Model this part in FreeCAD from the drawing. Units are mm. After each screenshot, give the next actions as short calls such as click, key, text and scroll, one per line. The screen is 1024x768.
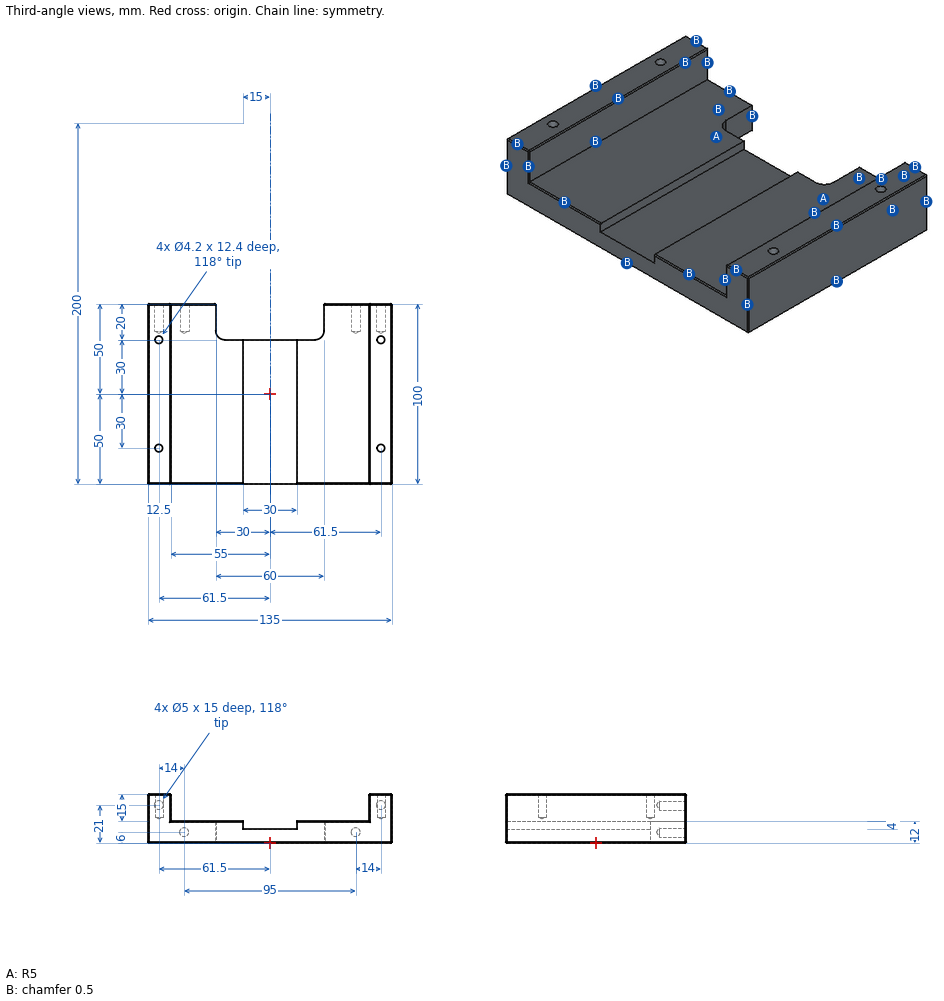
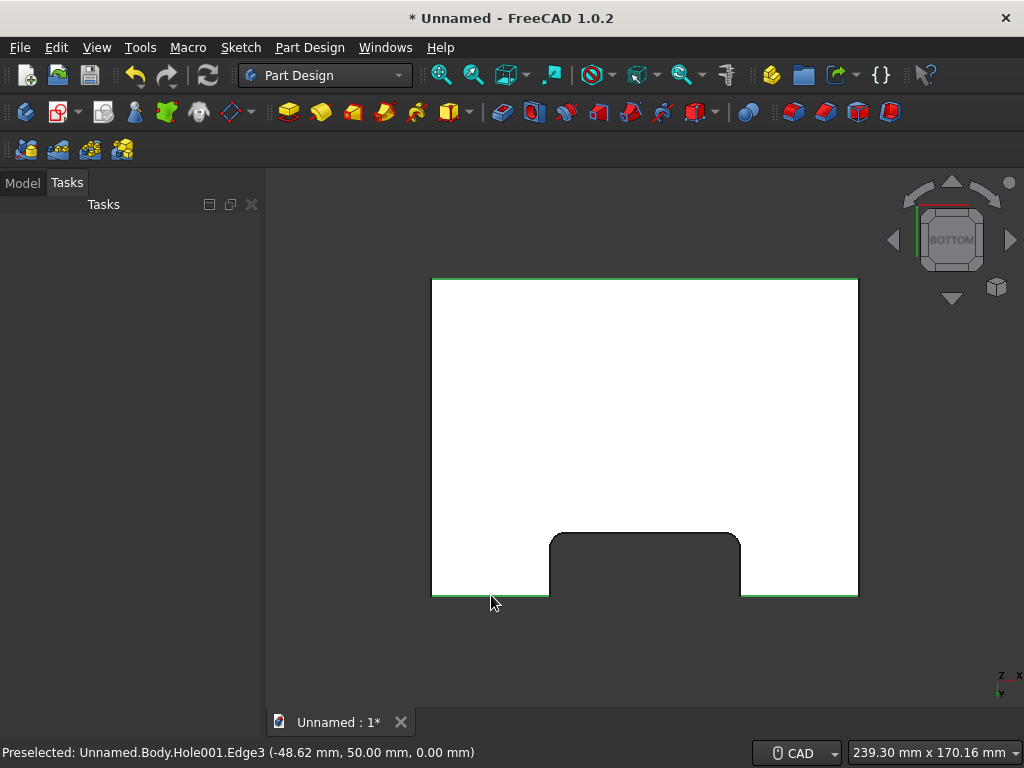
key(4)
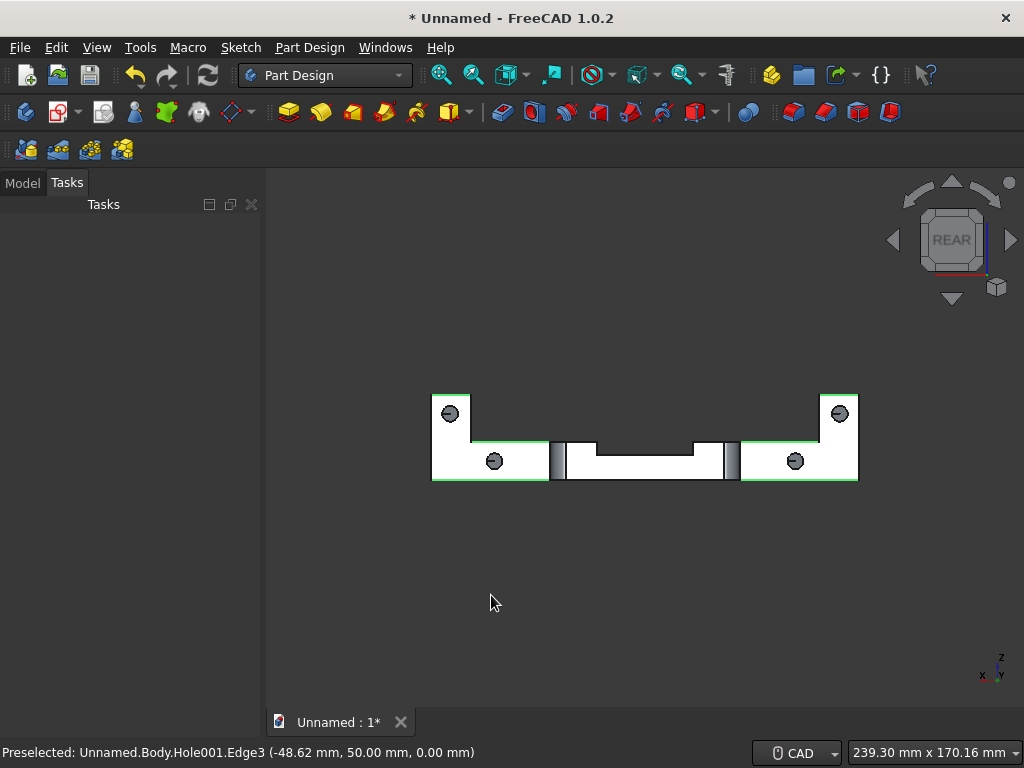
click(819, 417, ctrl)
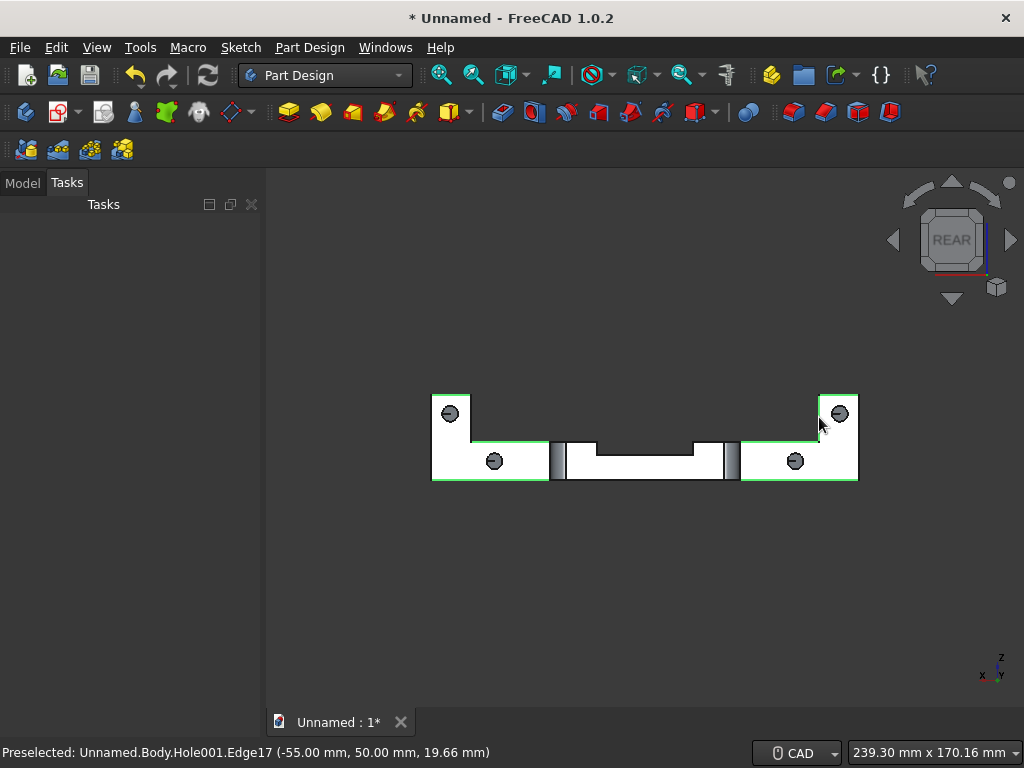
click(471, 417, ctrl)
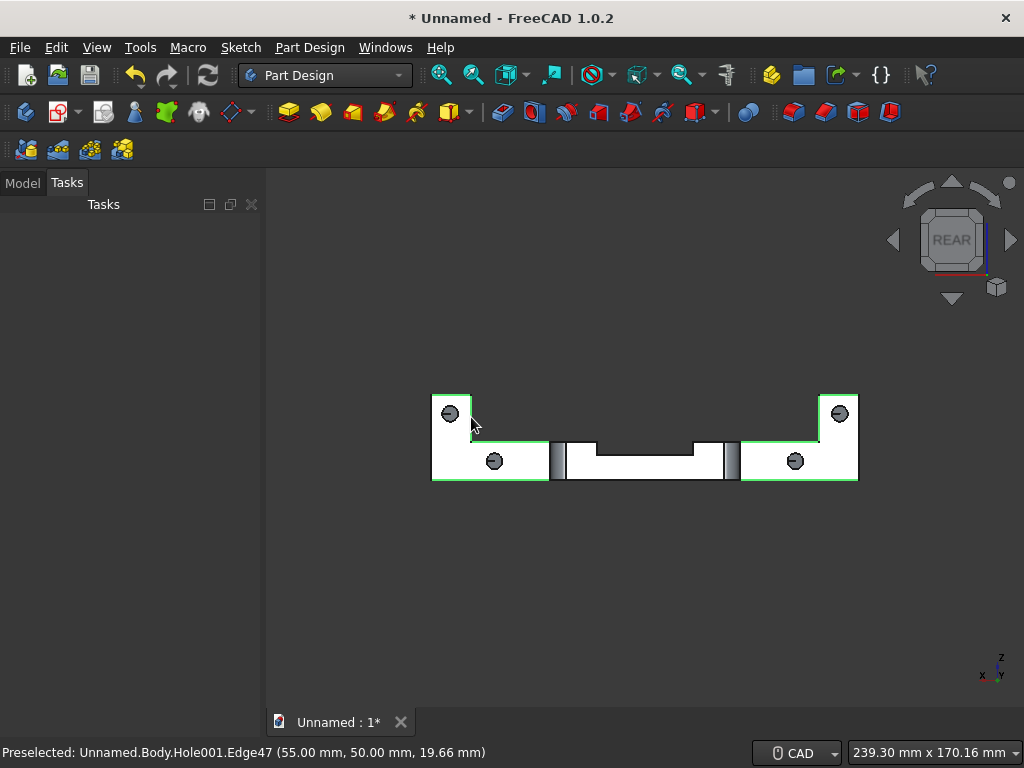
click(740, 460, ctrl)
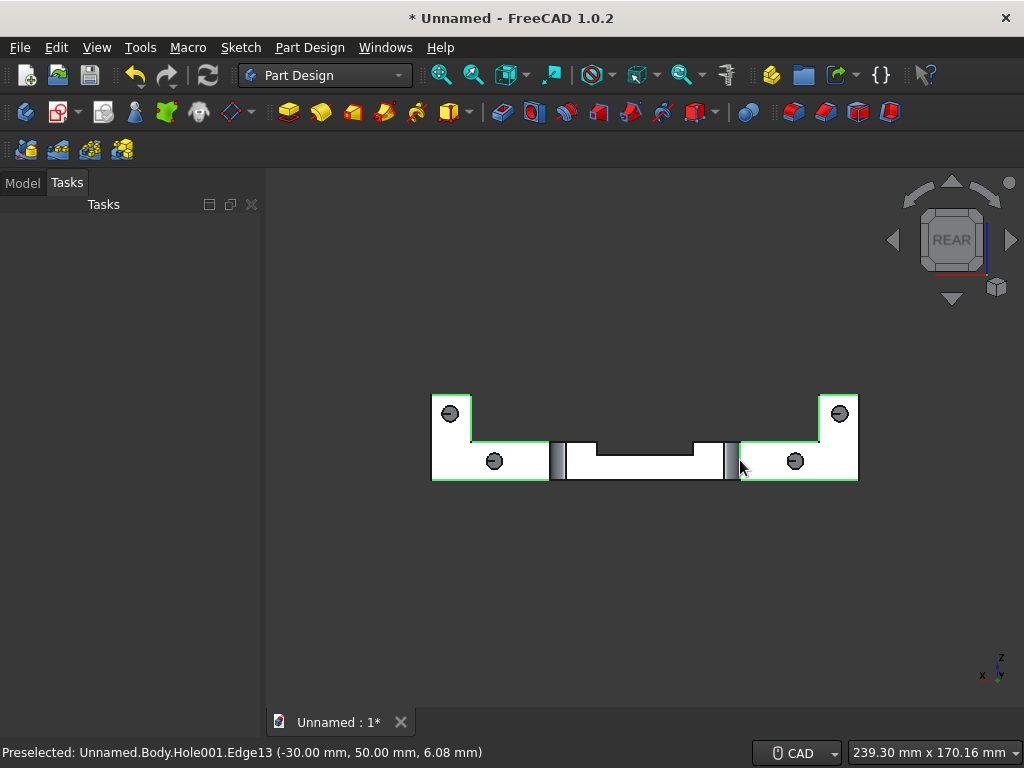
click(550, 460, ctrl)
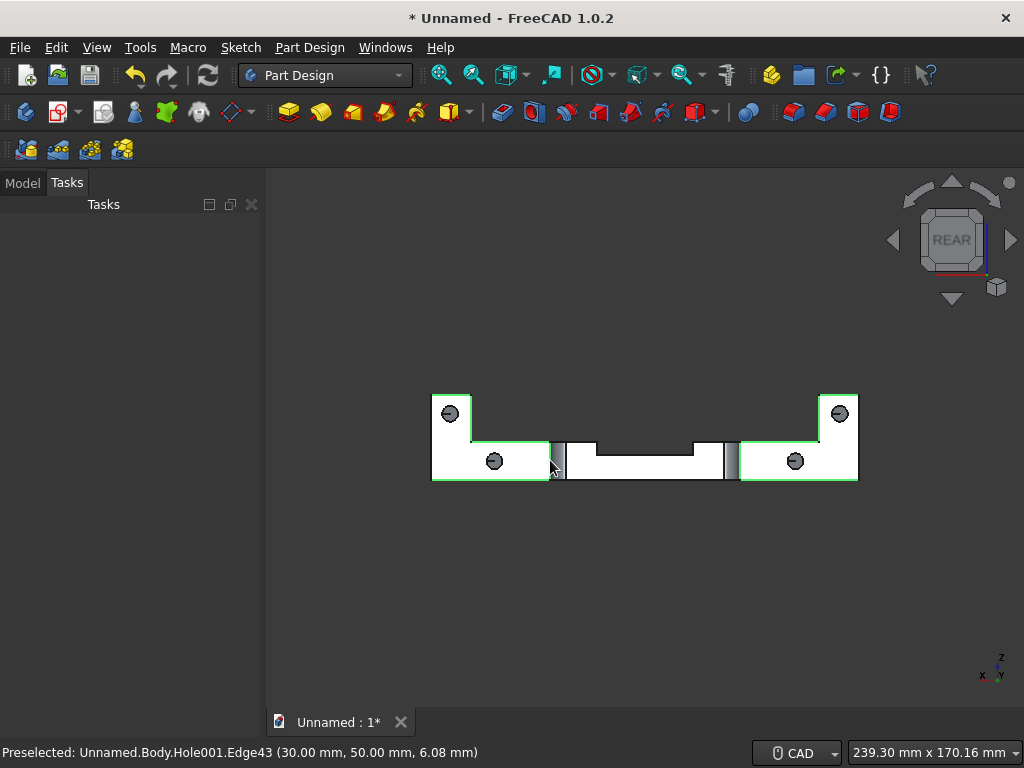
key(6)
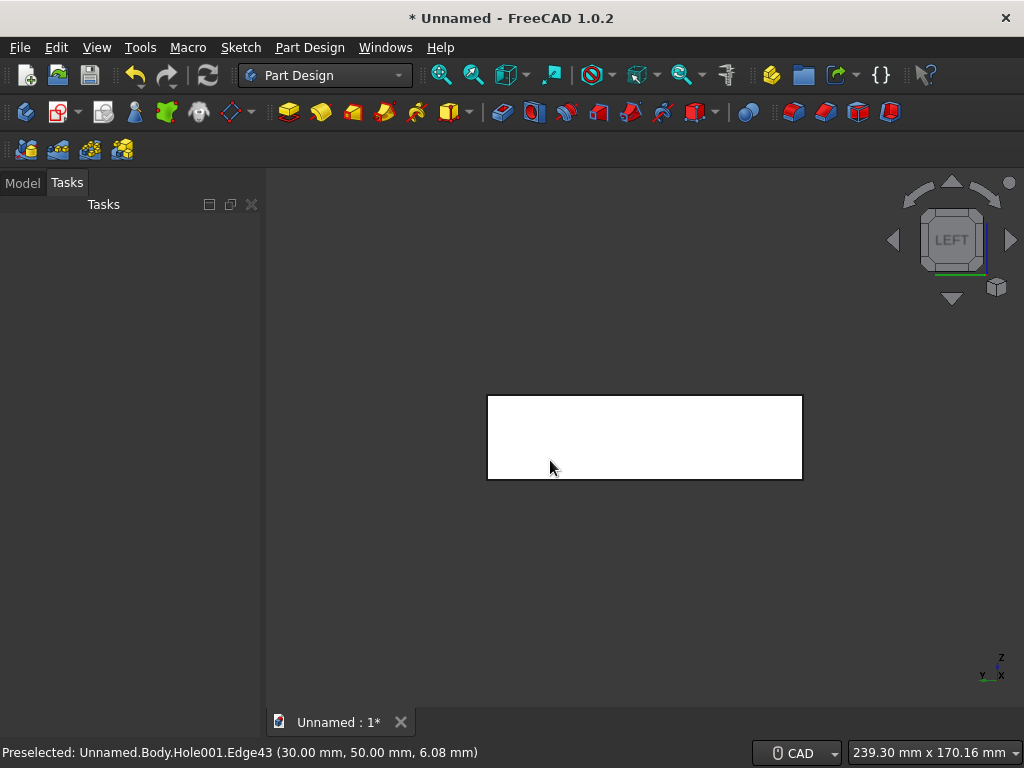
key(v)
key(f)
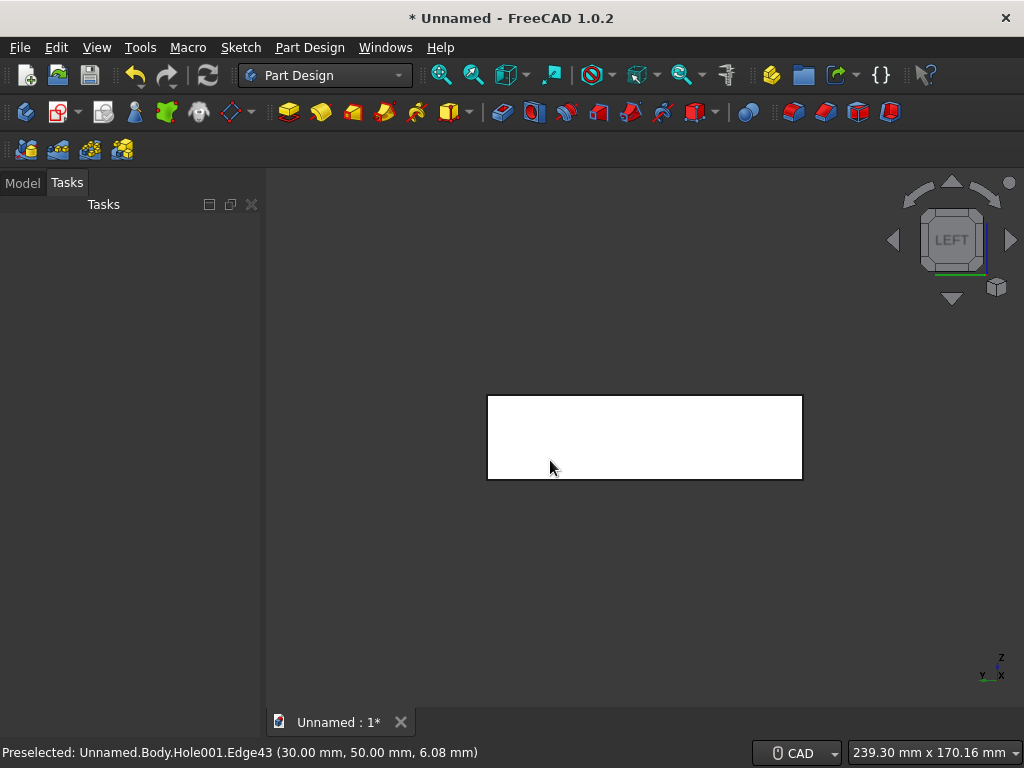
click(554, 436, ctrl)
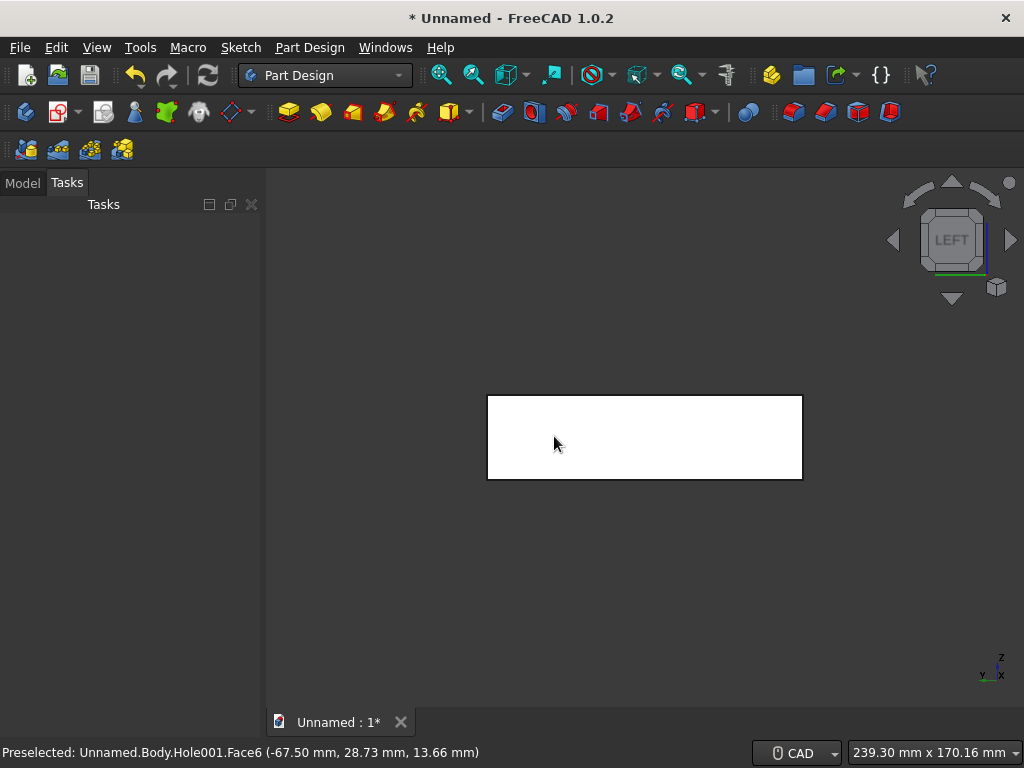
click(826, 112)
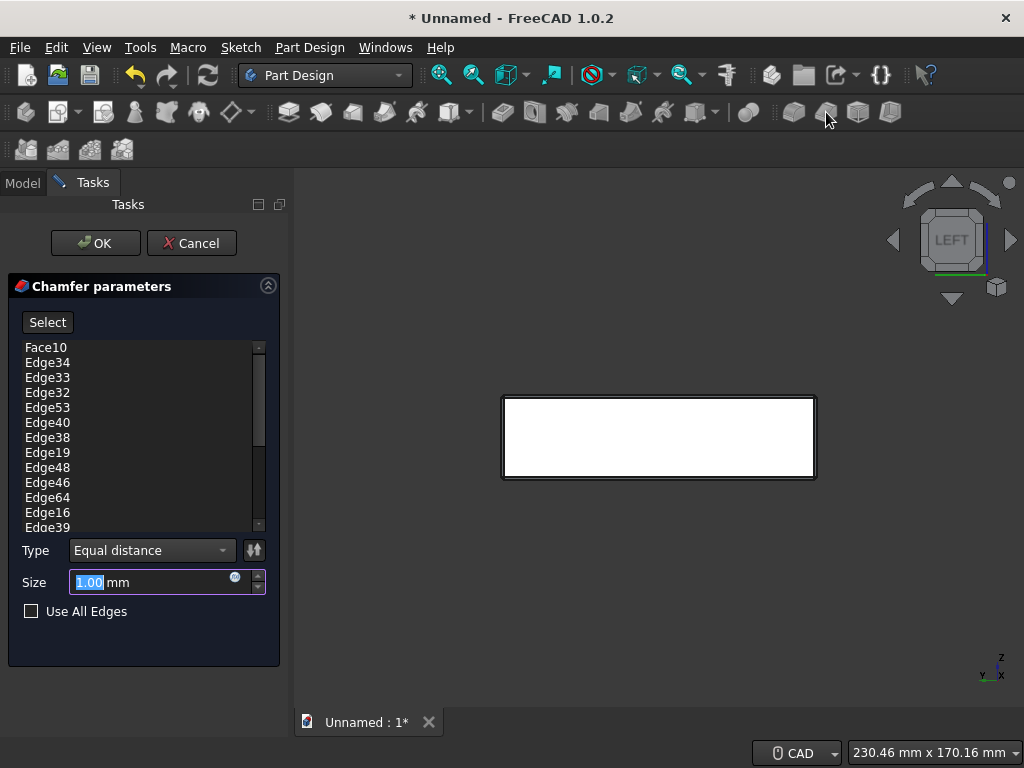
text(0.5)
key(Tab)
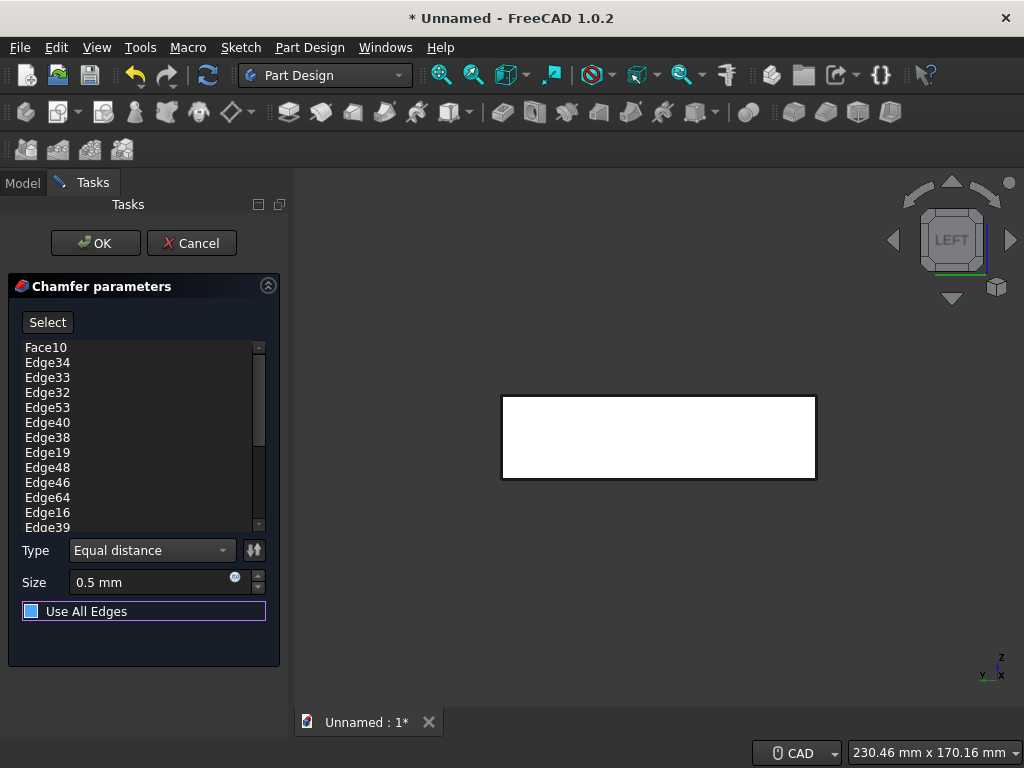
click(96, 243)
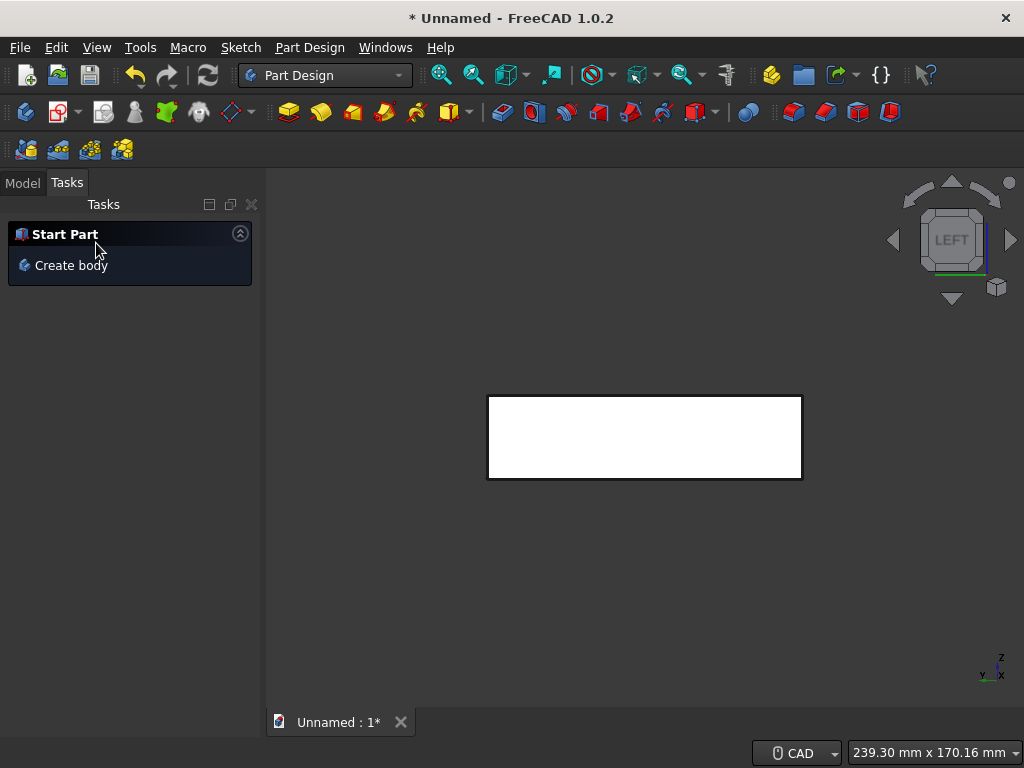
key(0)